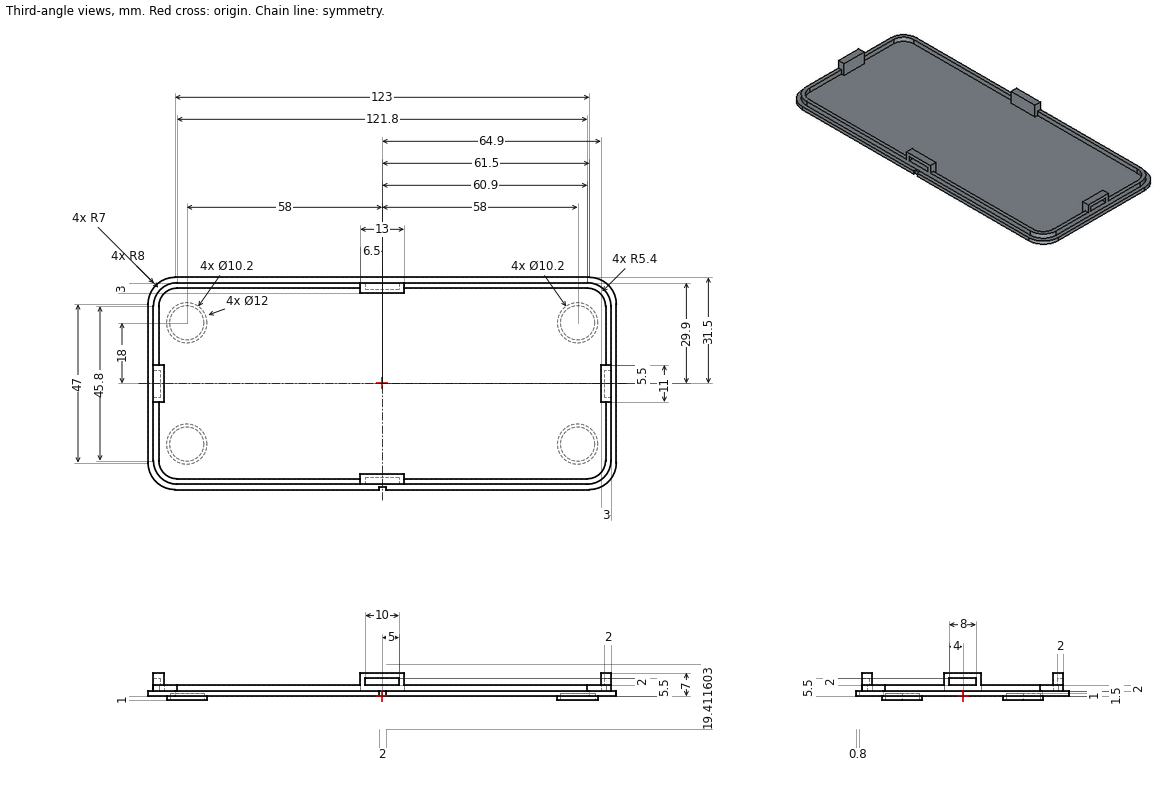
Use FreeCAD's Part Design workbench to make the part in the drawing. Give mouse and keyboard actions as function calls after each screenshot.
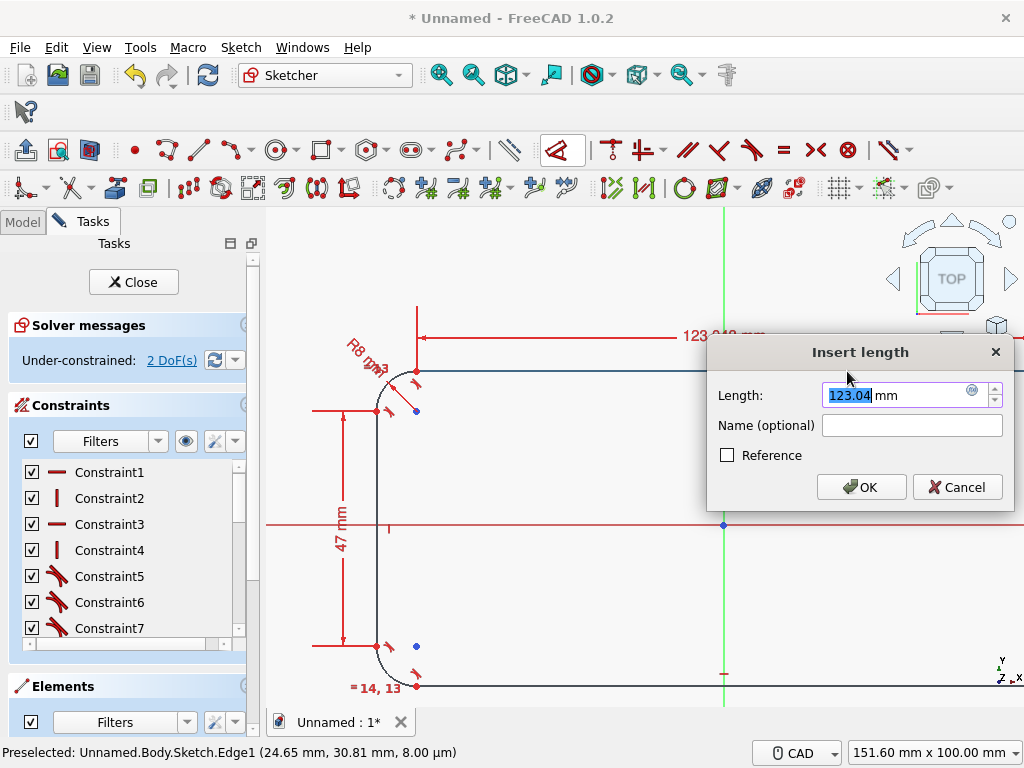
text(123)
key(Return)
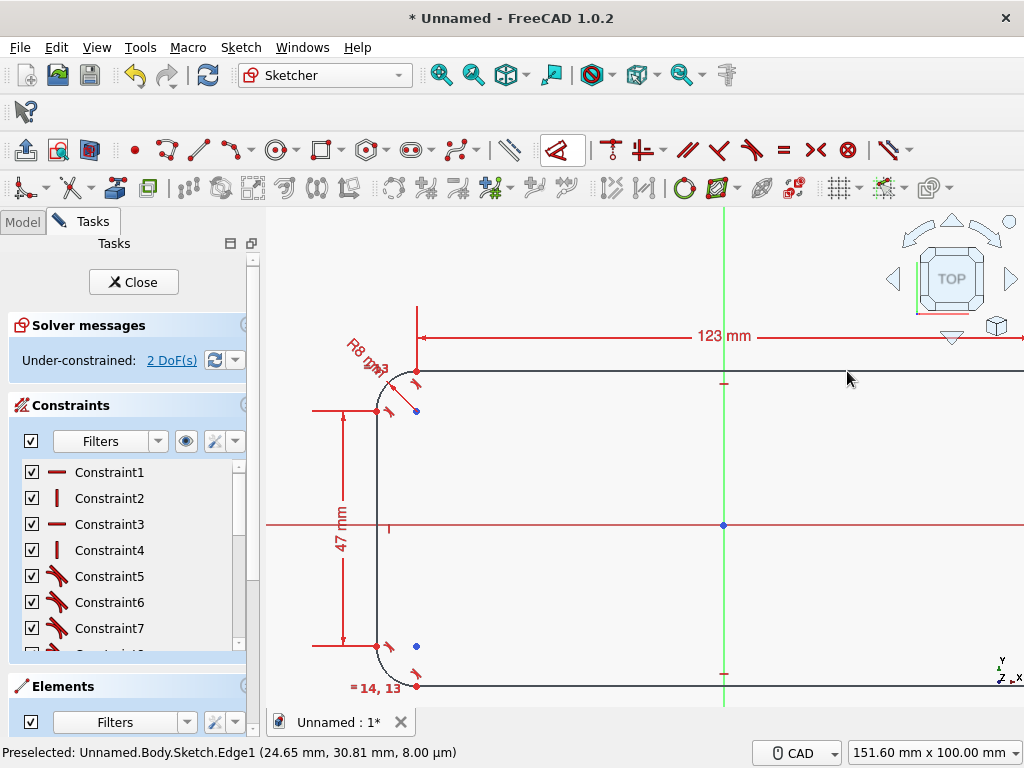
scroll(397, 374, down, 3)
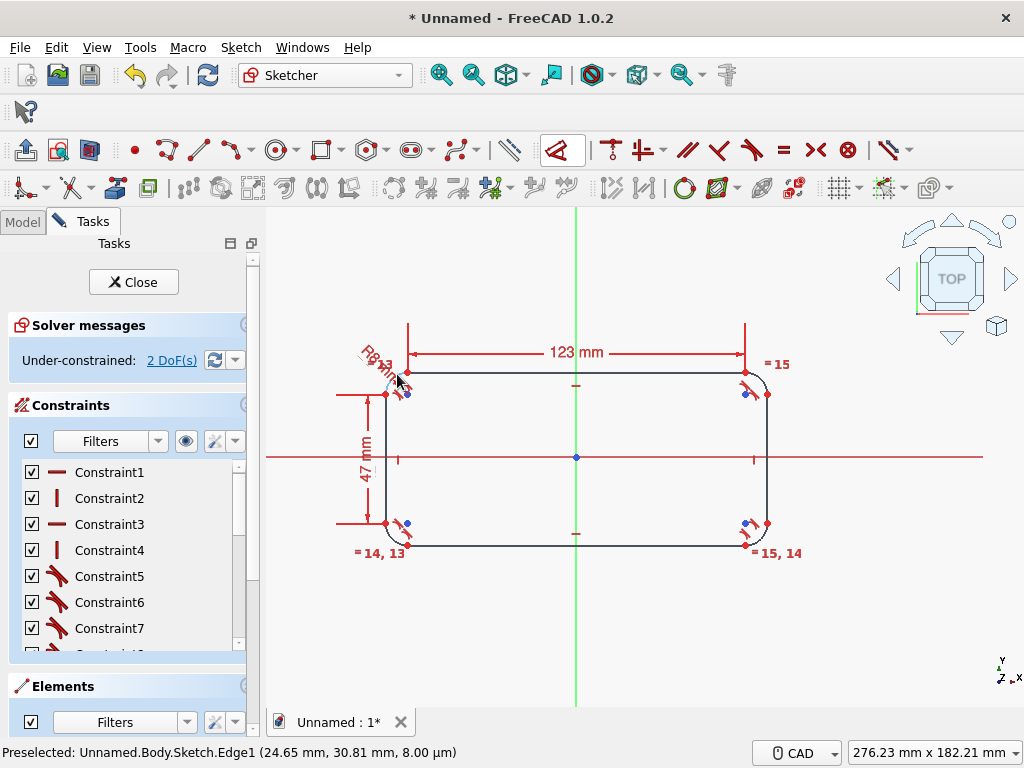
click(745, 373)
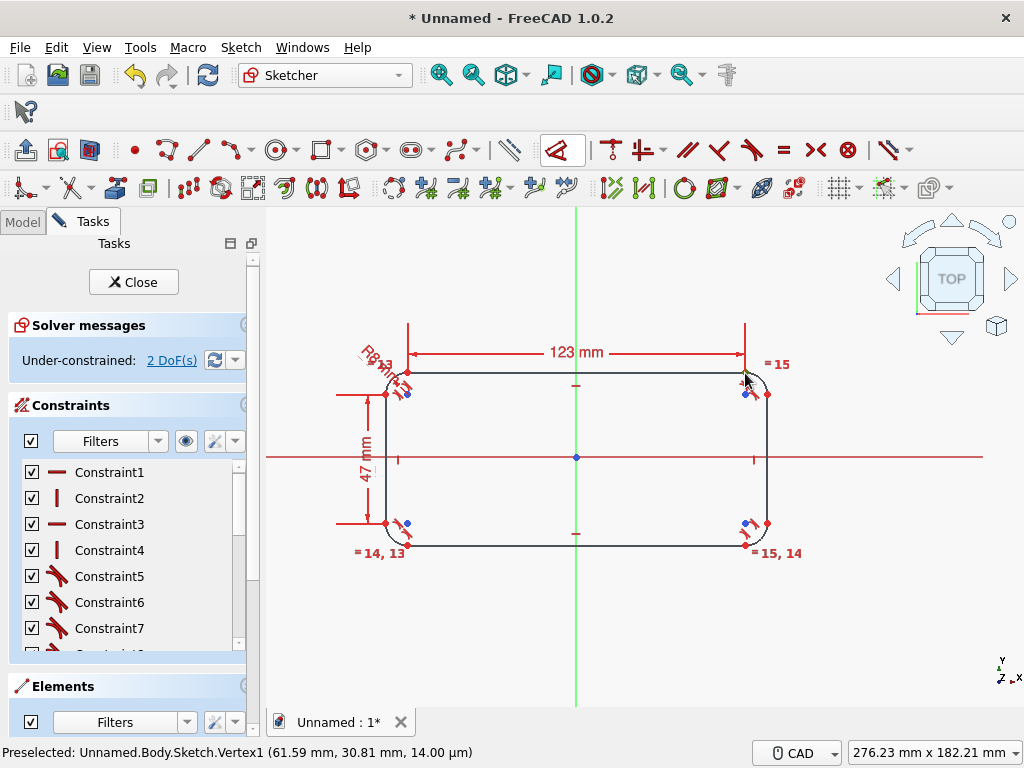
key(l)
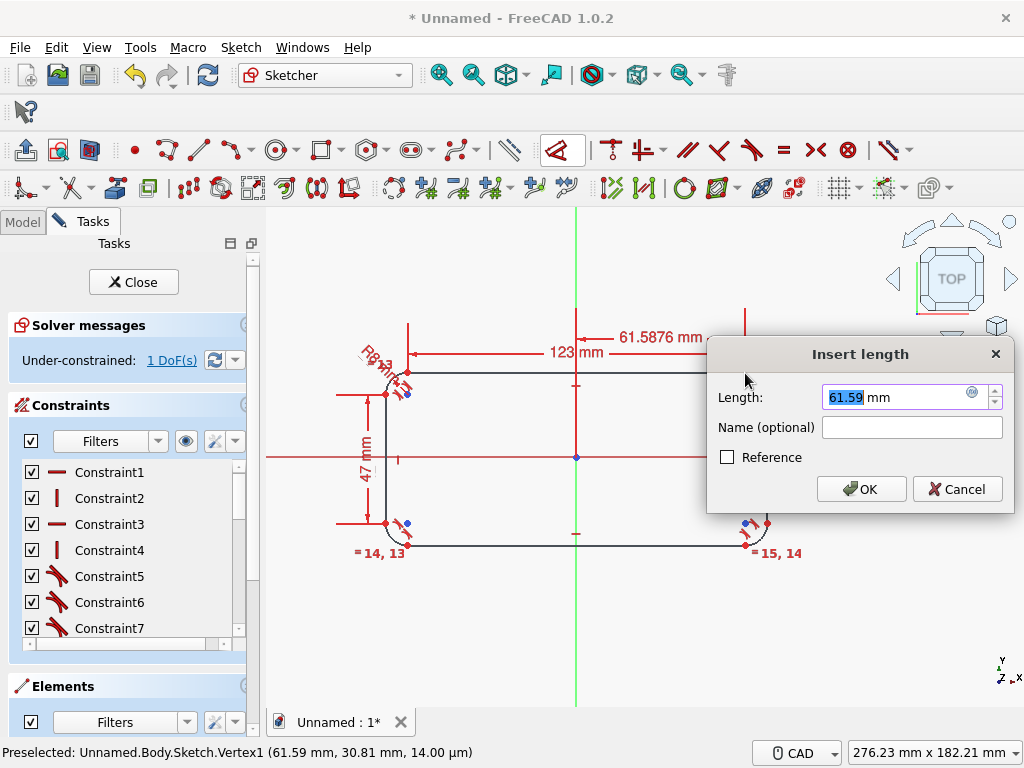
text(61.5)
key(Return)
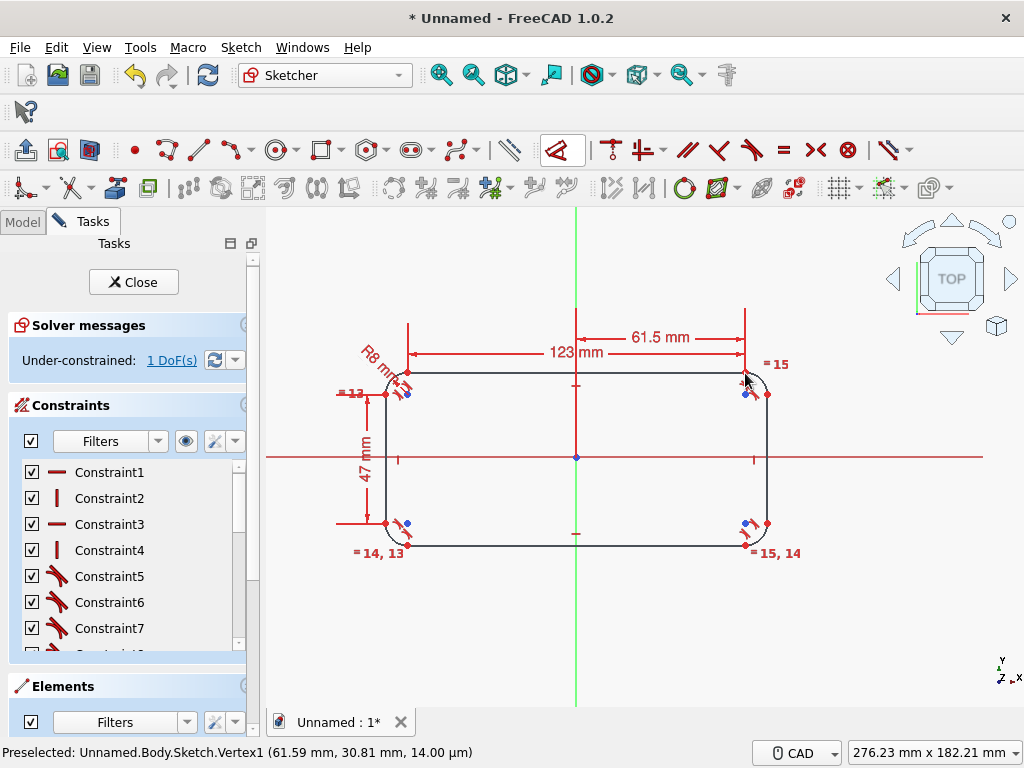
click(745, 373)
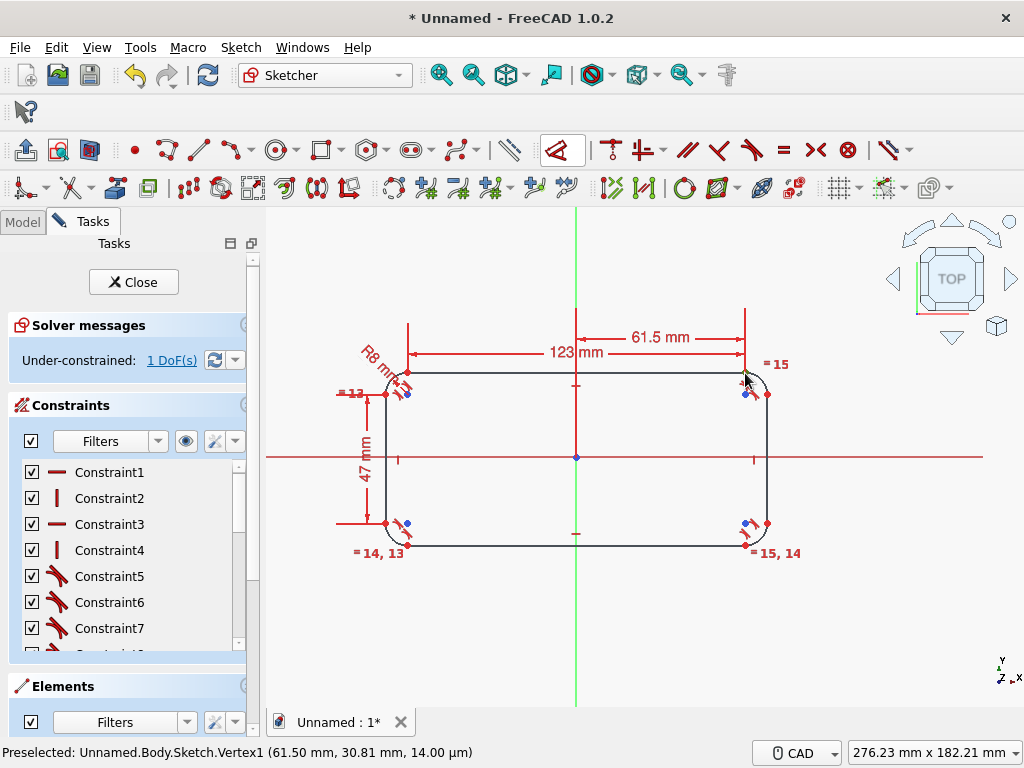
key(i)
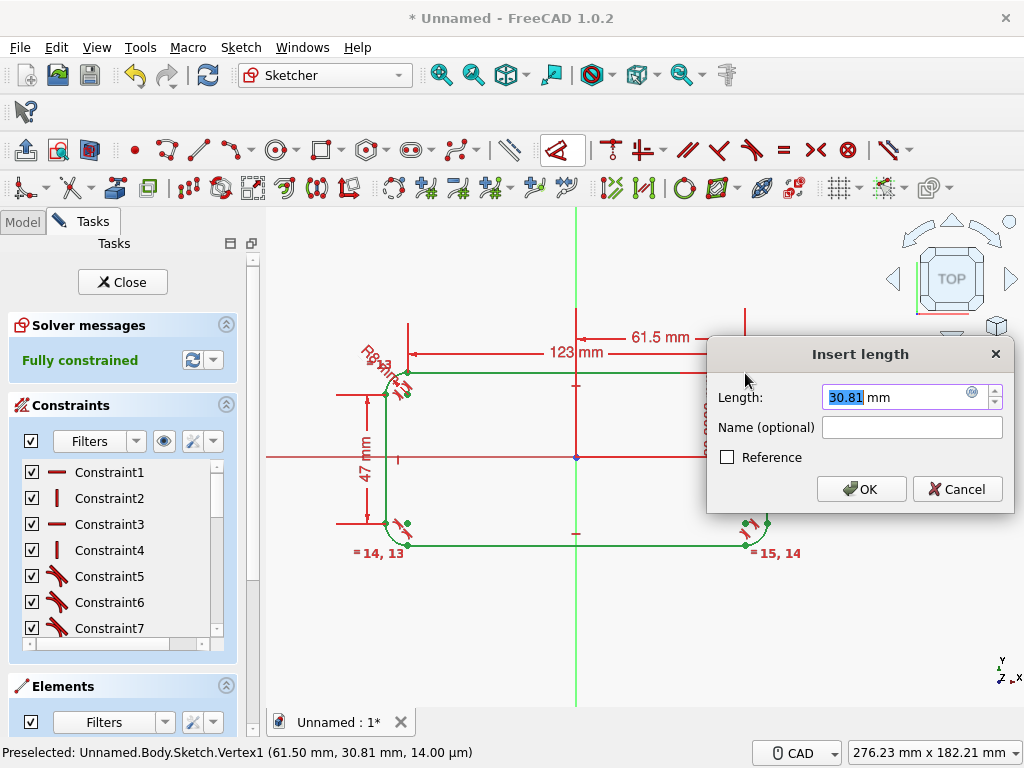
text(31.5)
key(Return)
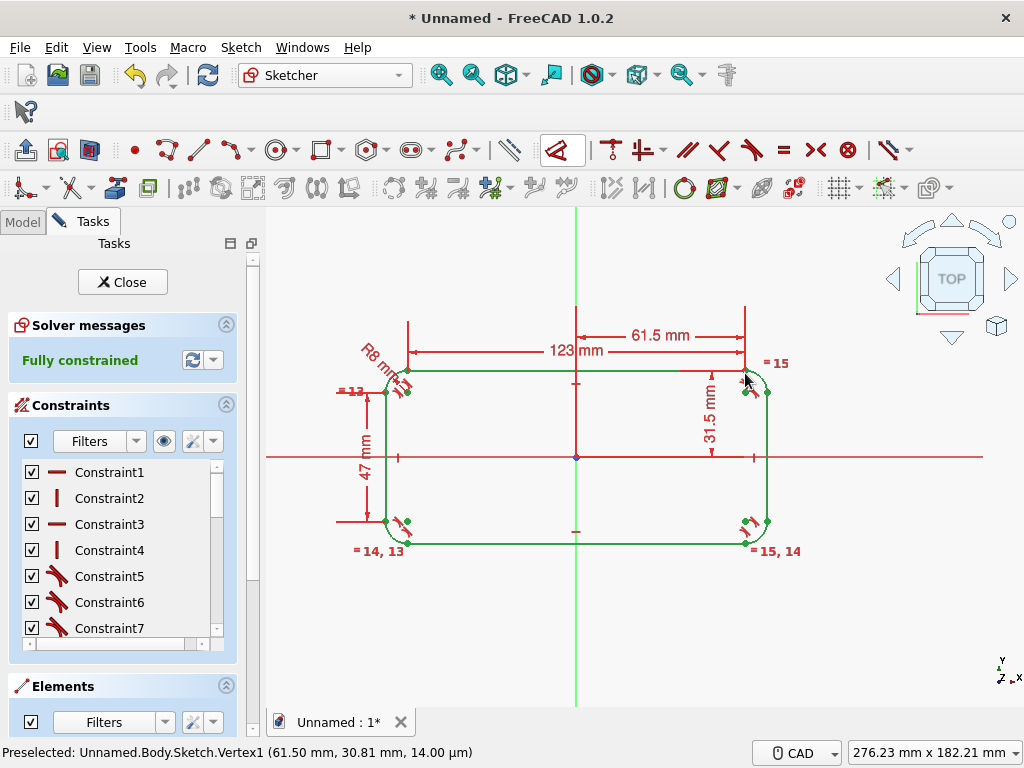
click(123, 282)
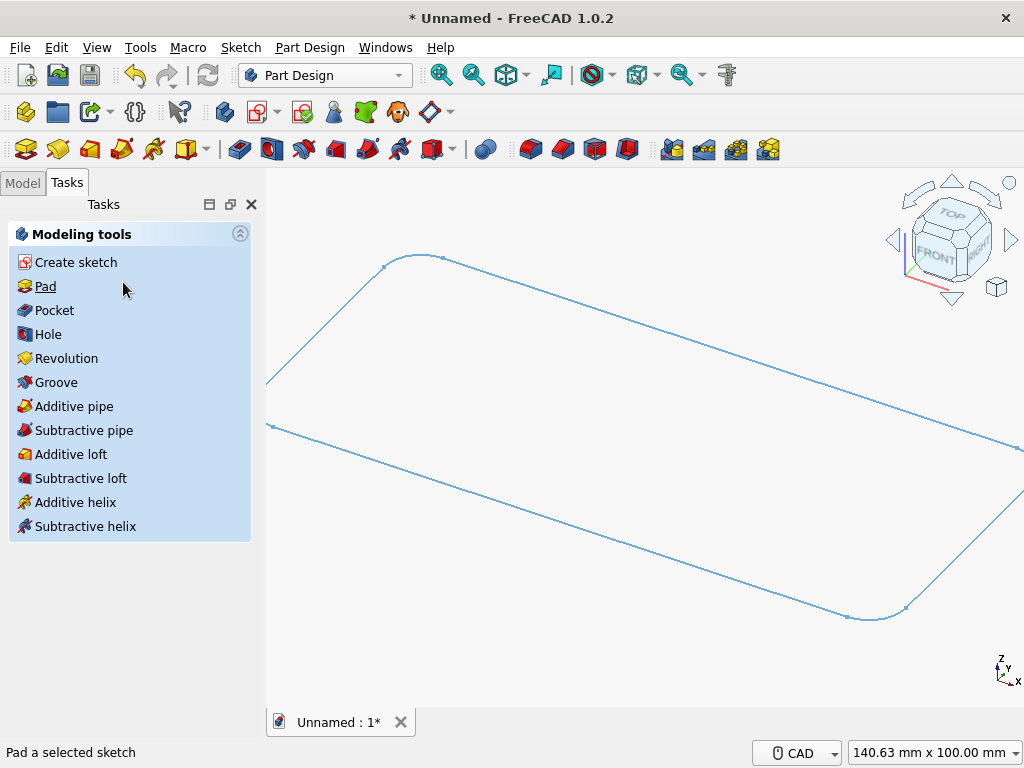
click(26, 150)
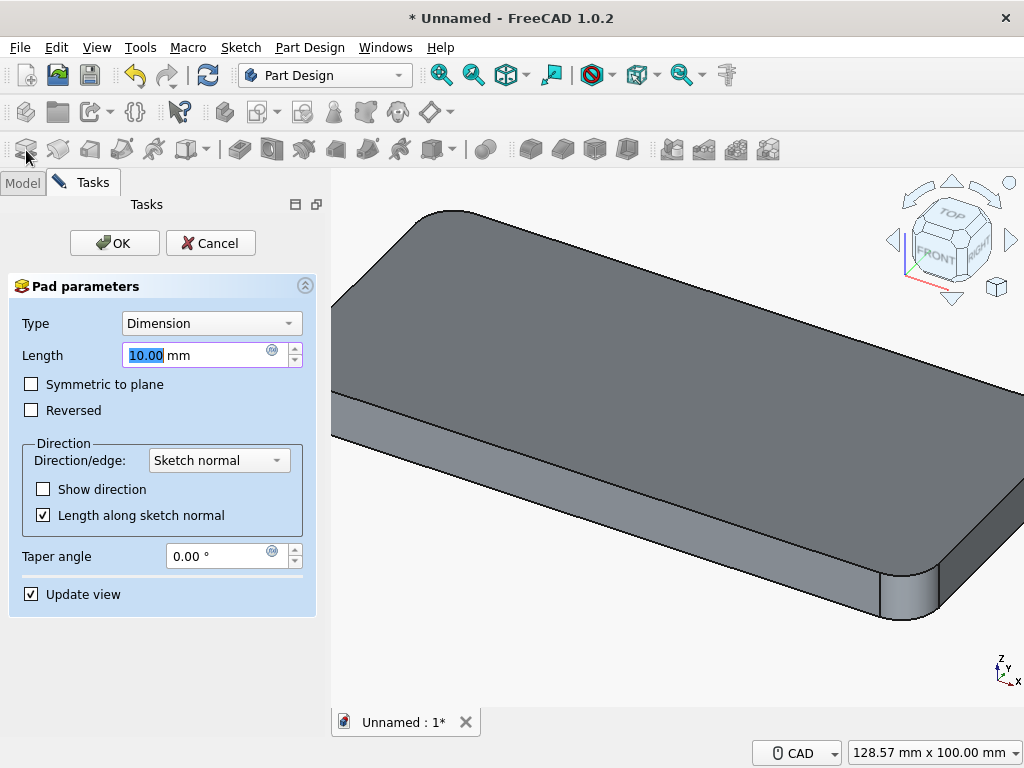
text(1.5)
key(Tab)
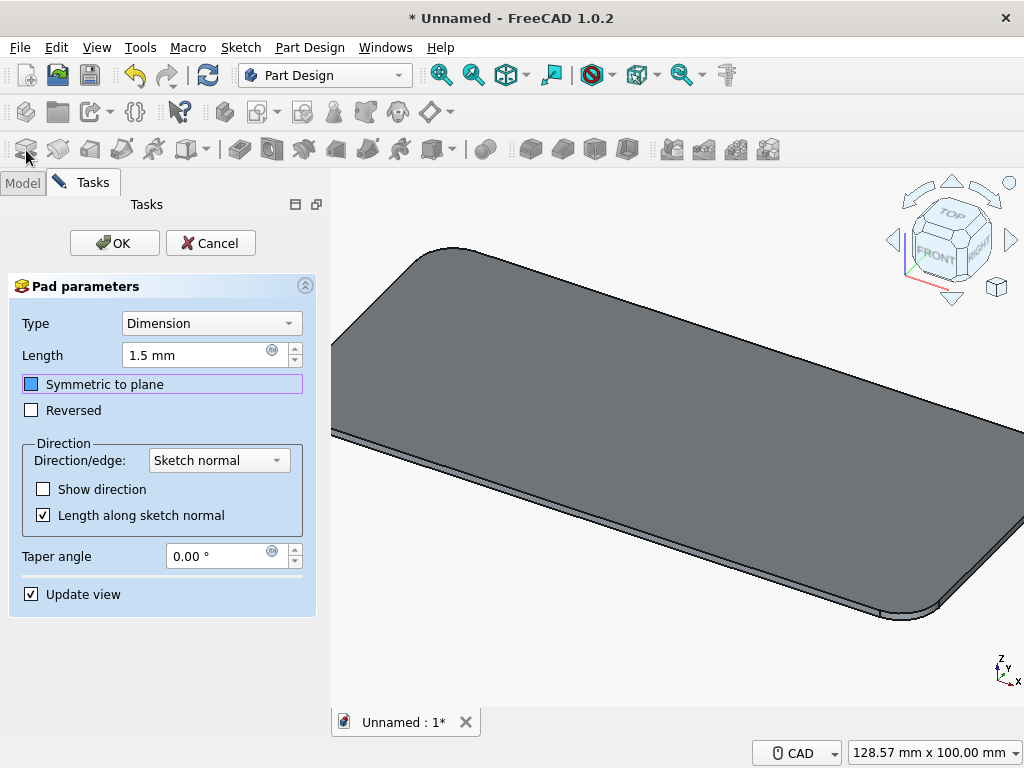
click(115, 243)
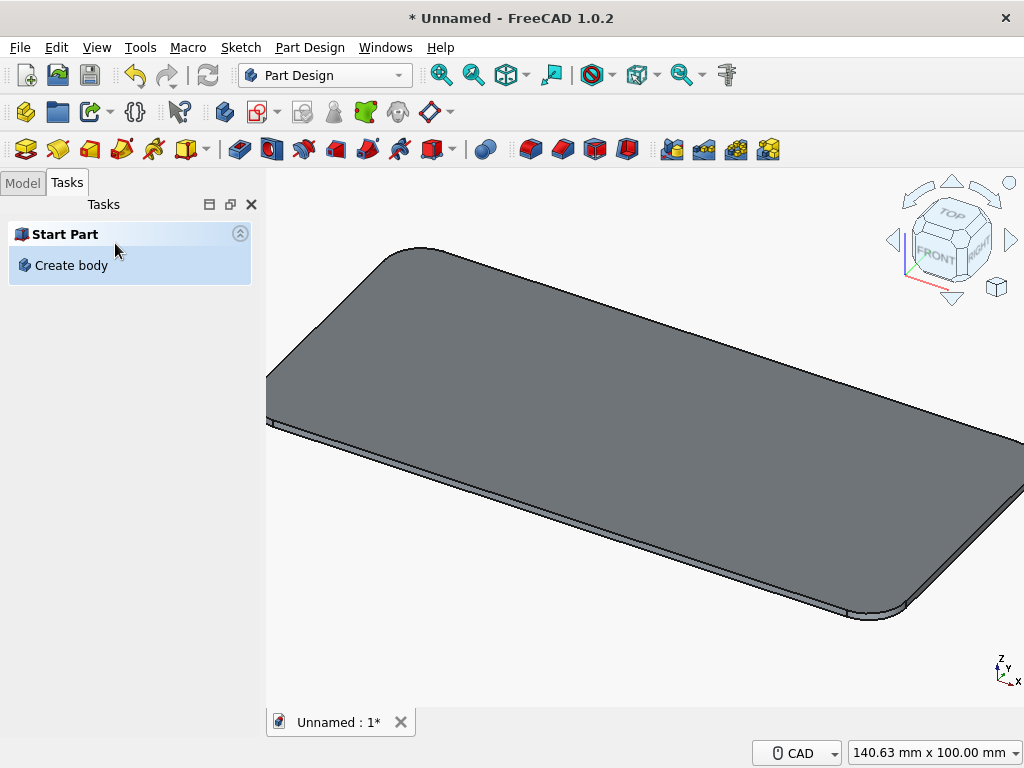
click(442, 76)